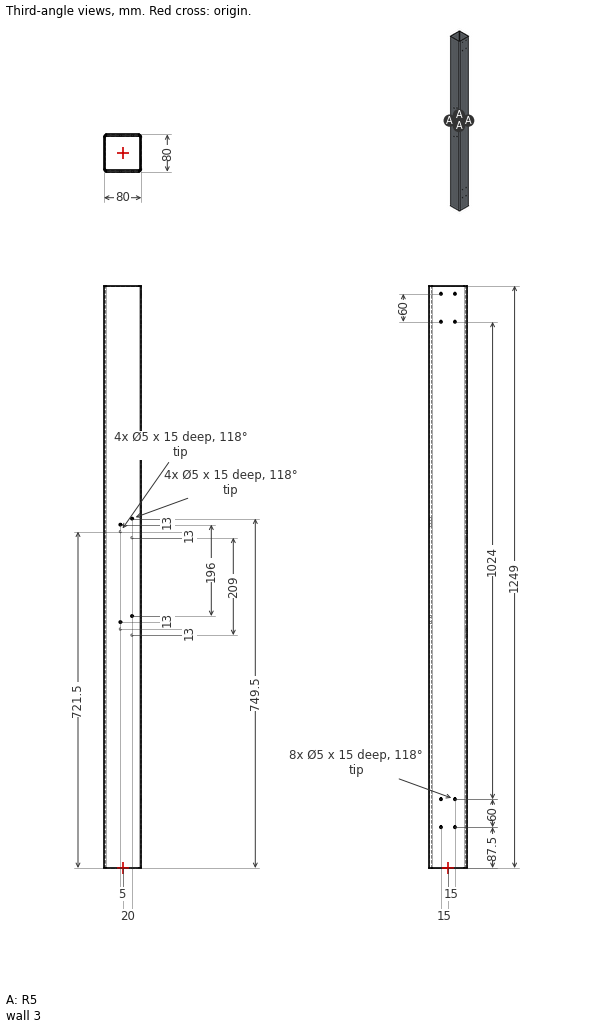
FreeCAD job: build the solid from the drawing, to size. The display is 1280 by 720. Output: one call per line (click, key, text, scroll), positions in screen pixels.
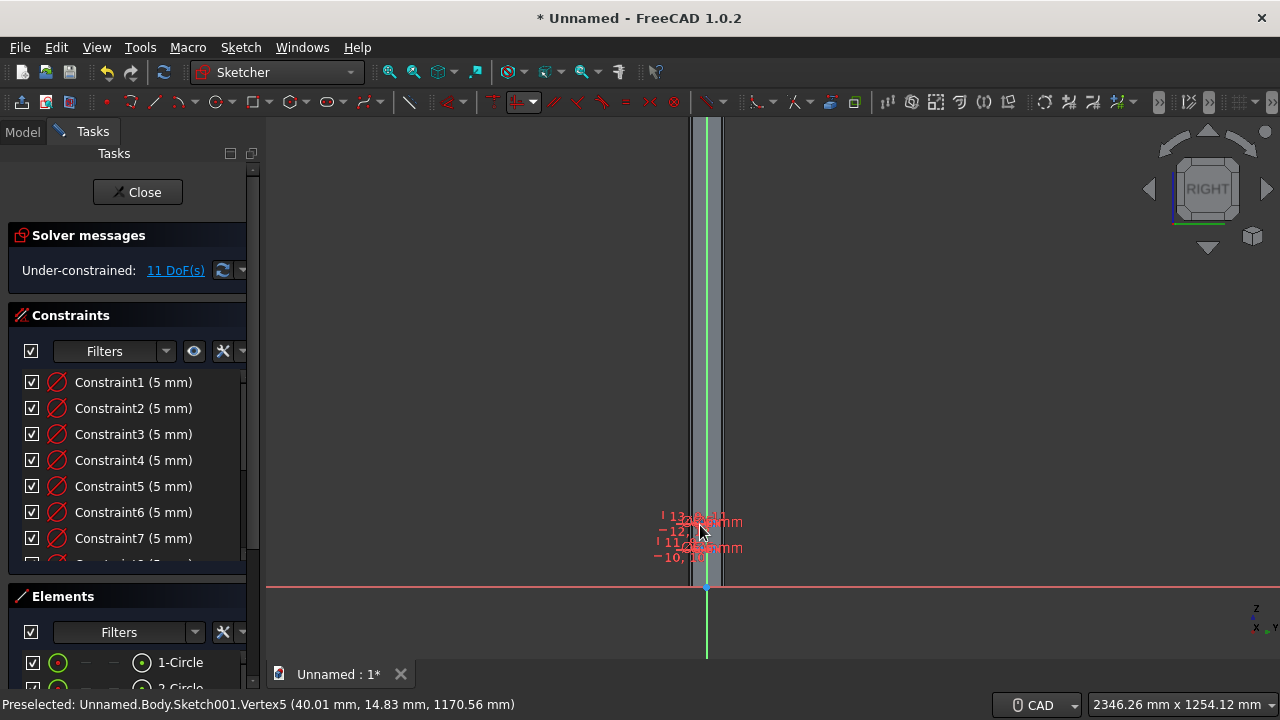
click(700, 524)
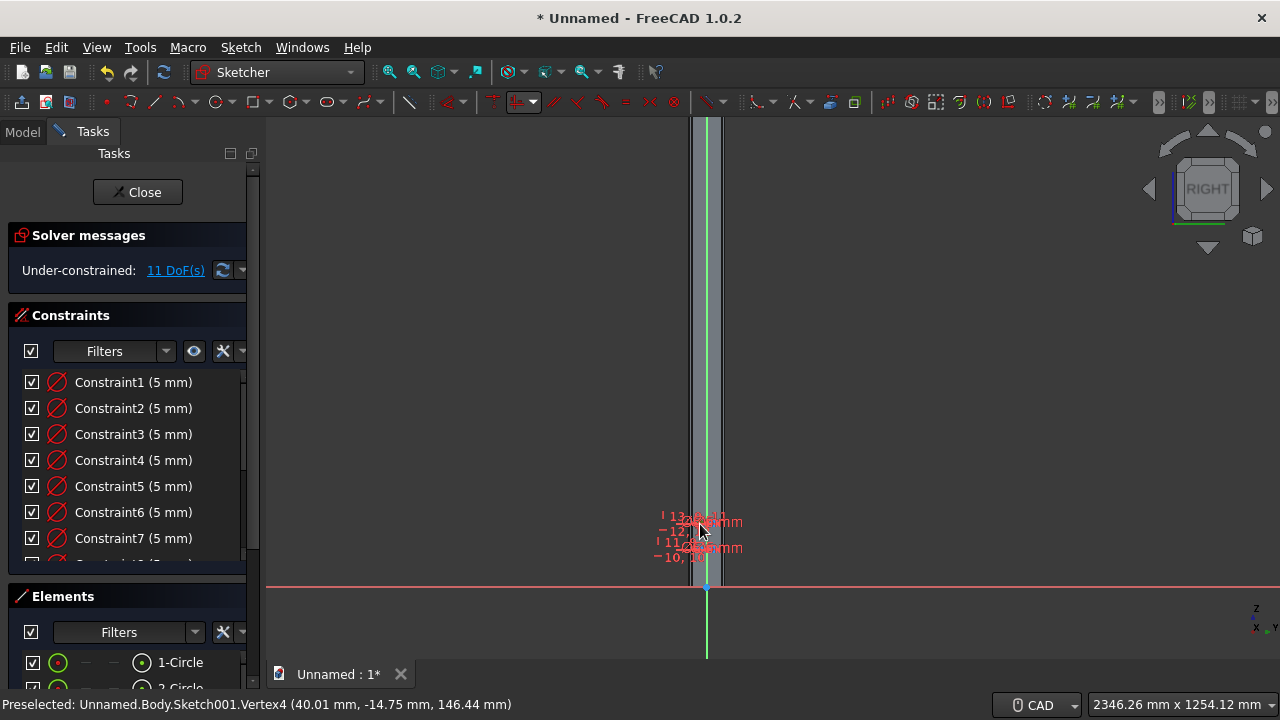
scroll(700, 525, down, 2)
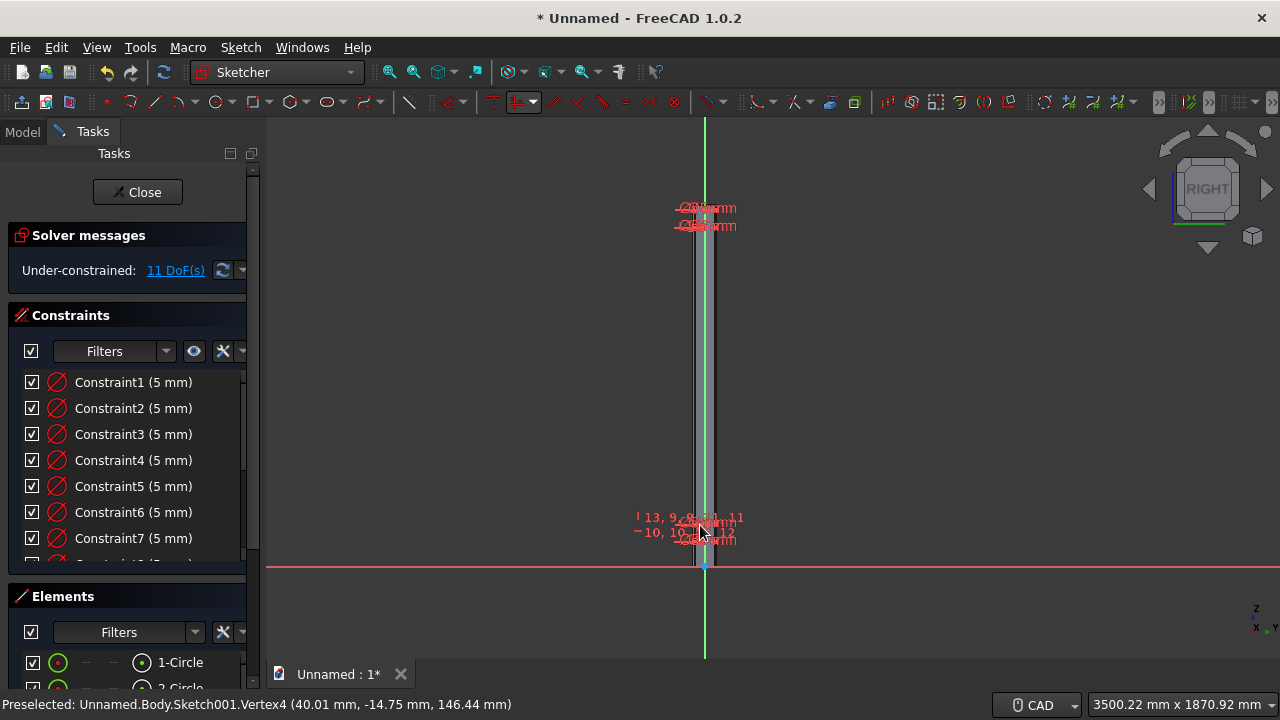
scroll(700, 228, up, 2)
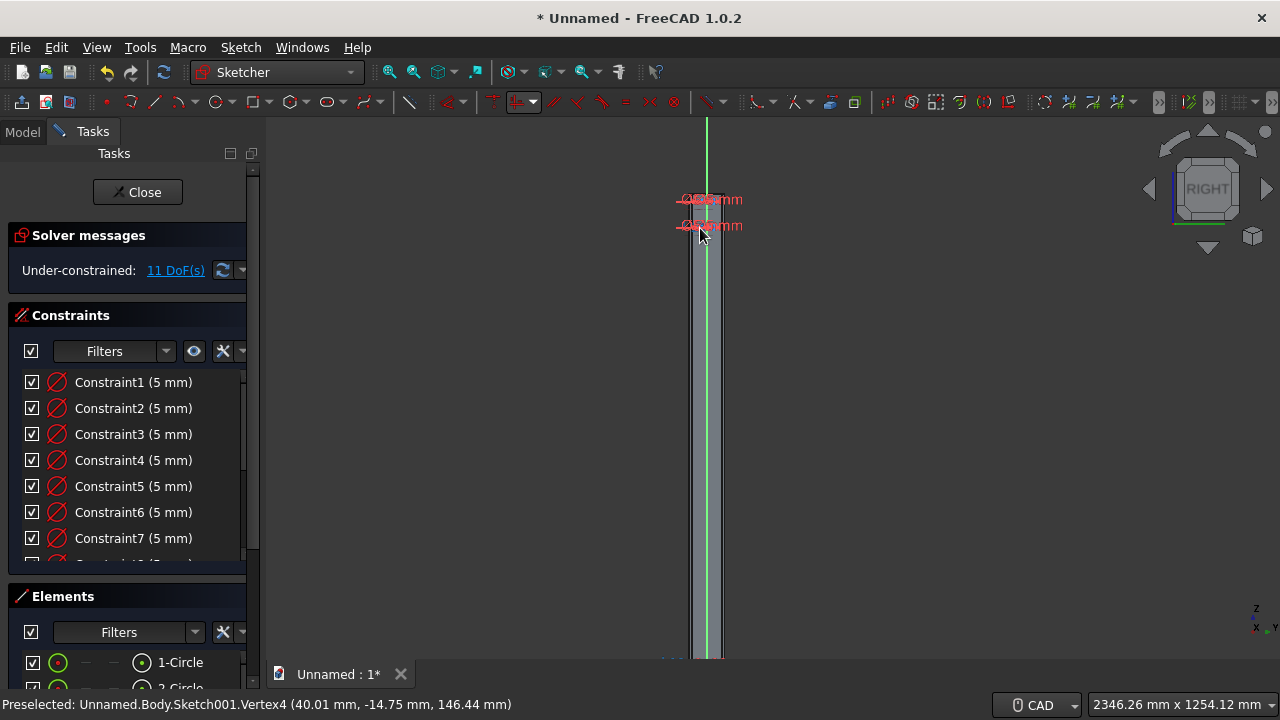
scroll(700, 228, up, 4)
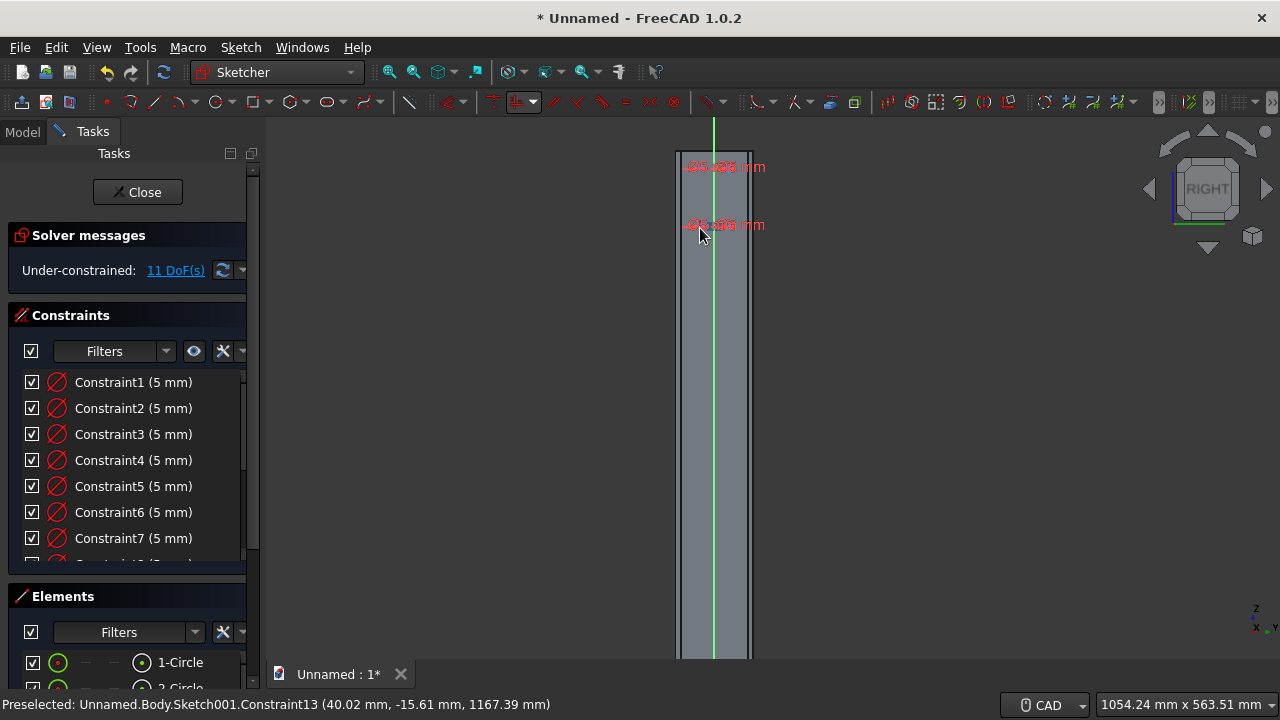
scroll(700, 227, up, 4)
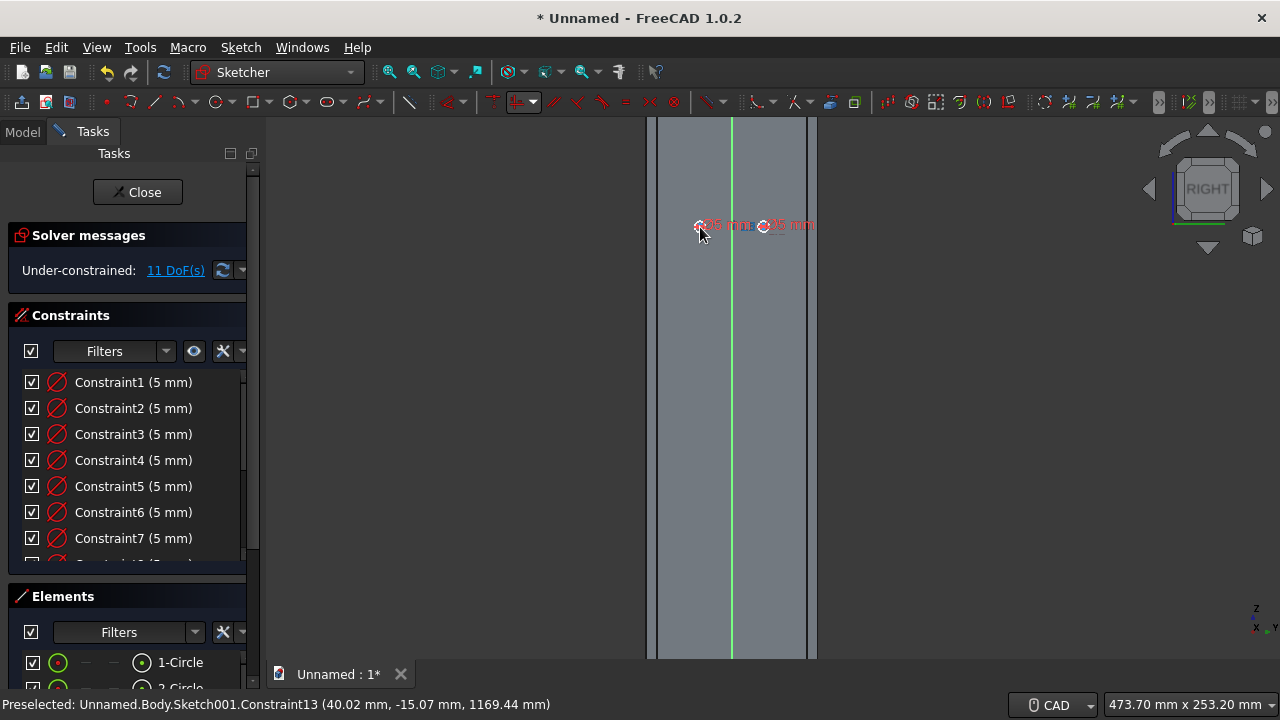
click(700, 227)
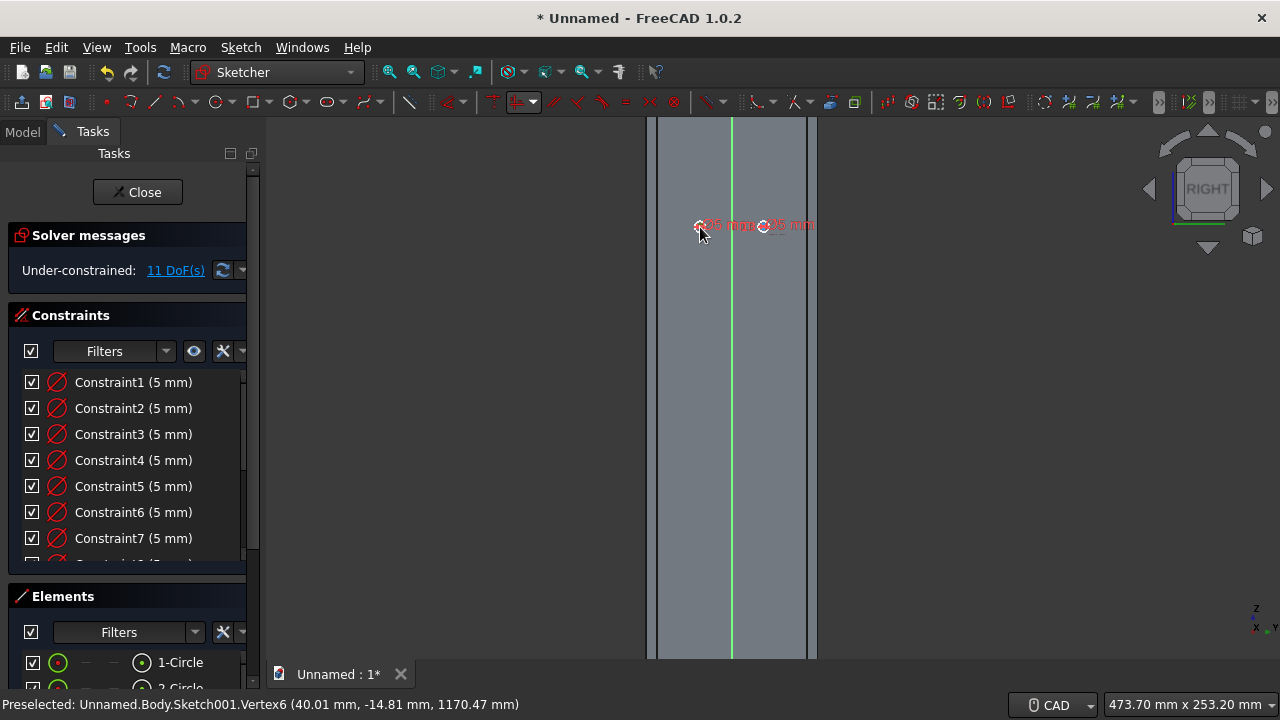
key(v)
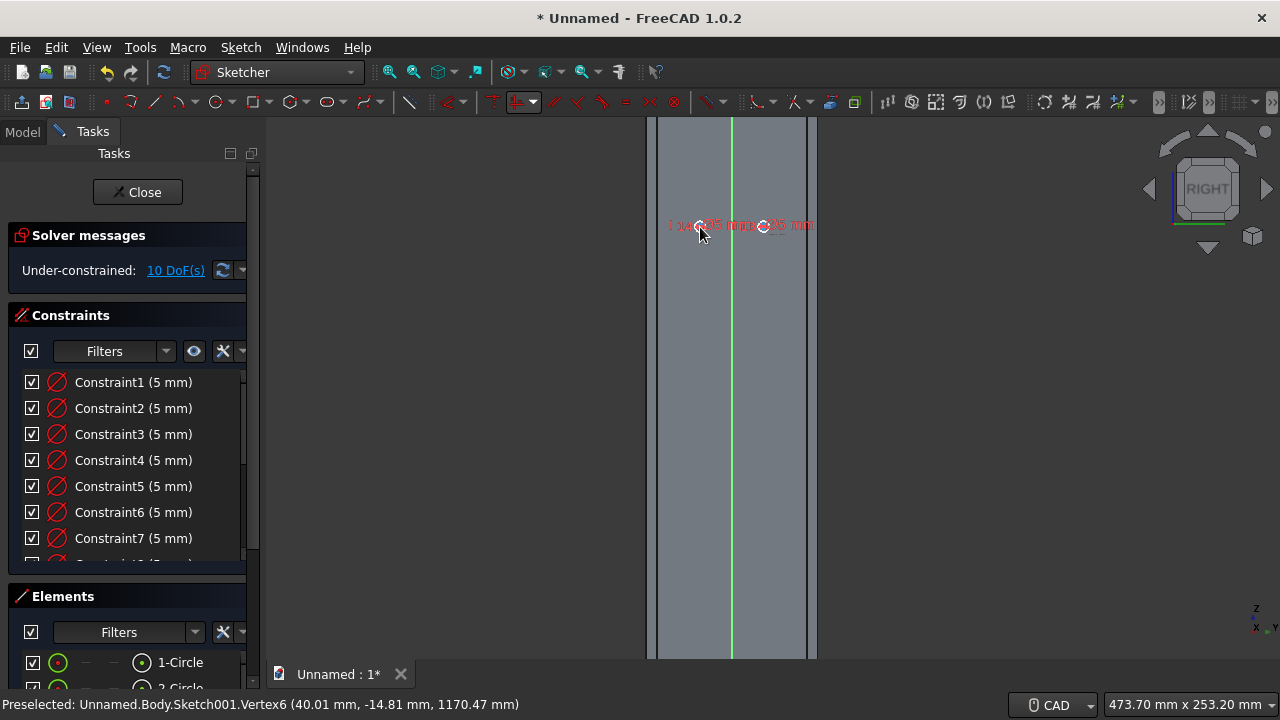
scroll(700, 228, down, 10)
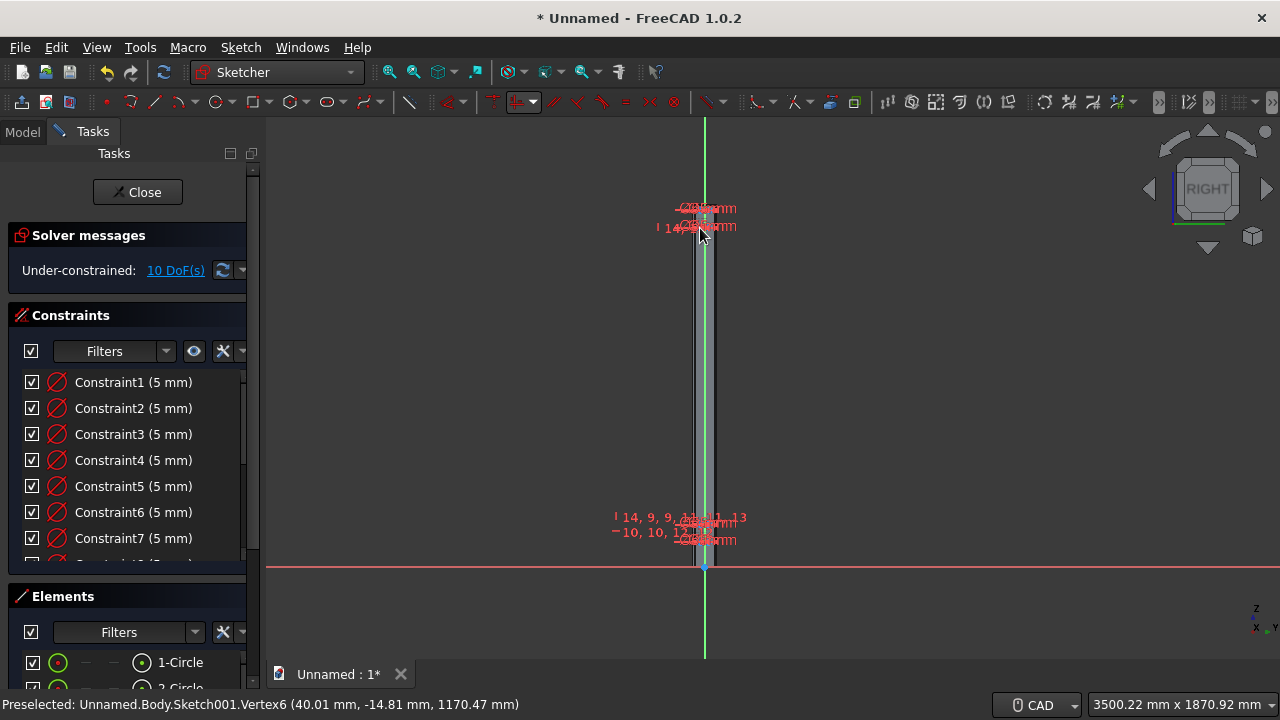
scroll(709, 228, up, 2)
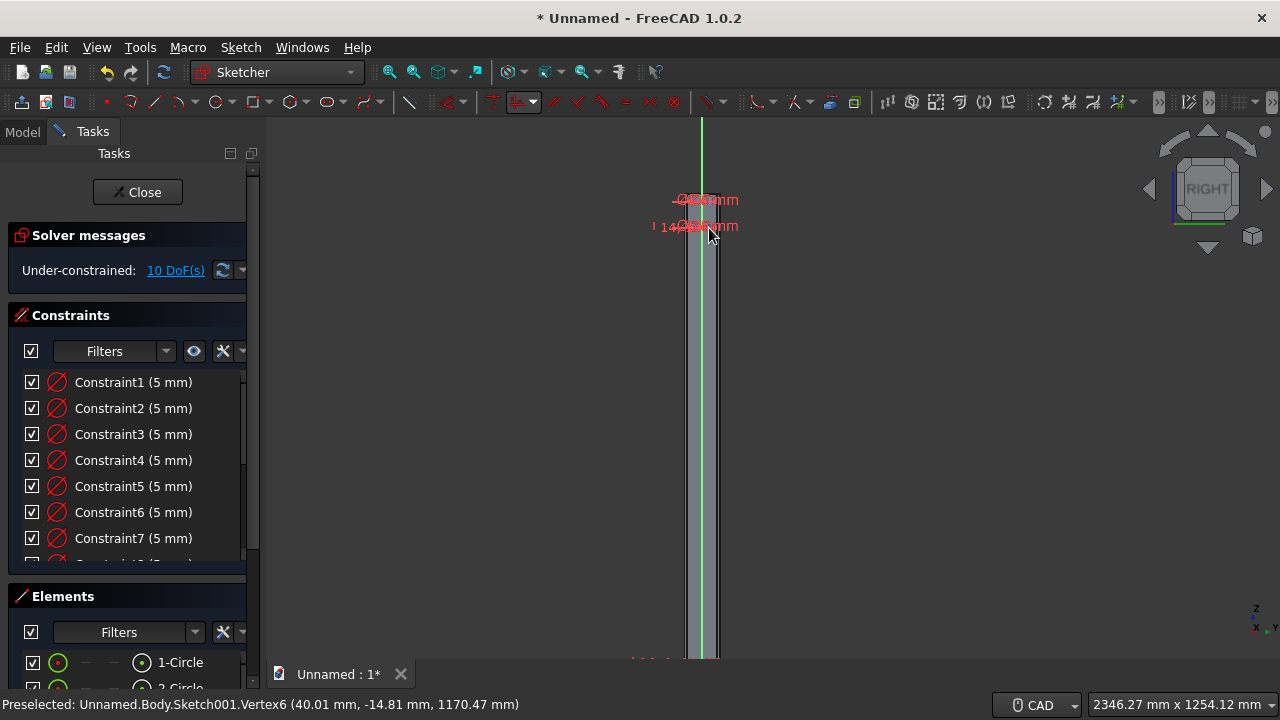
click(709, 228)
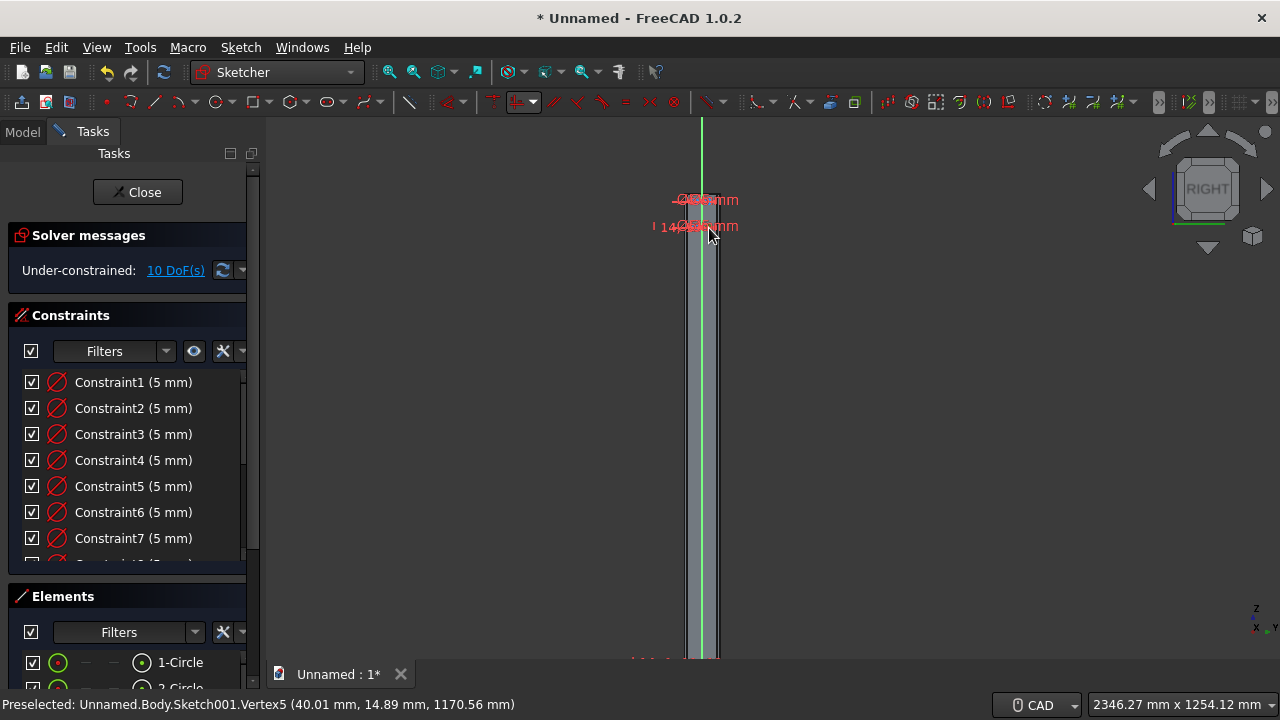
scroll(696, 228, up, 4)